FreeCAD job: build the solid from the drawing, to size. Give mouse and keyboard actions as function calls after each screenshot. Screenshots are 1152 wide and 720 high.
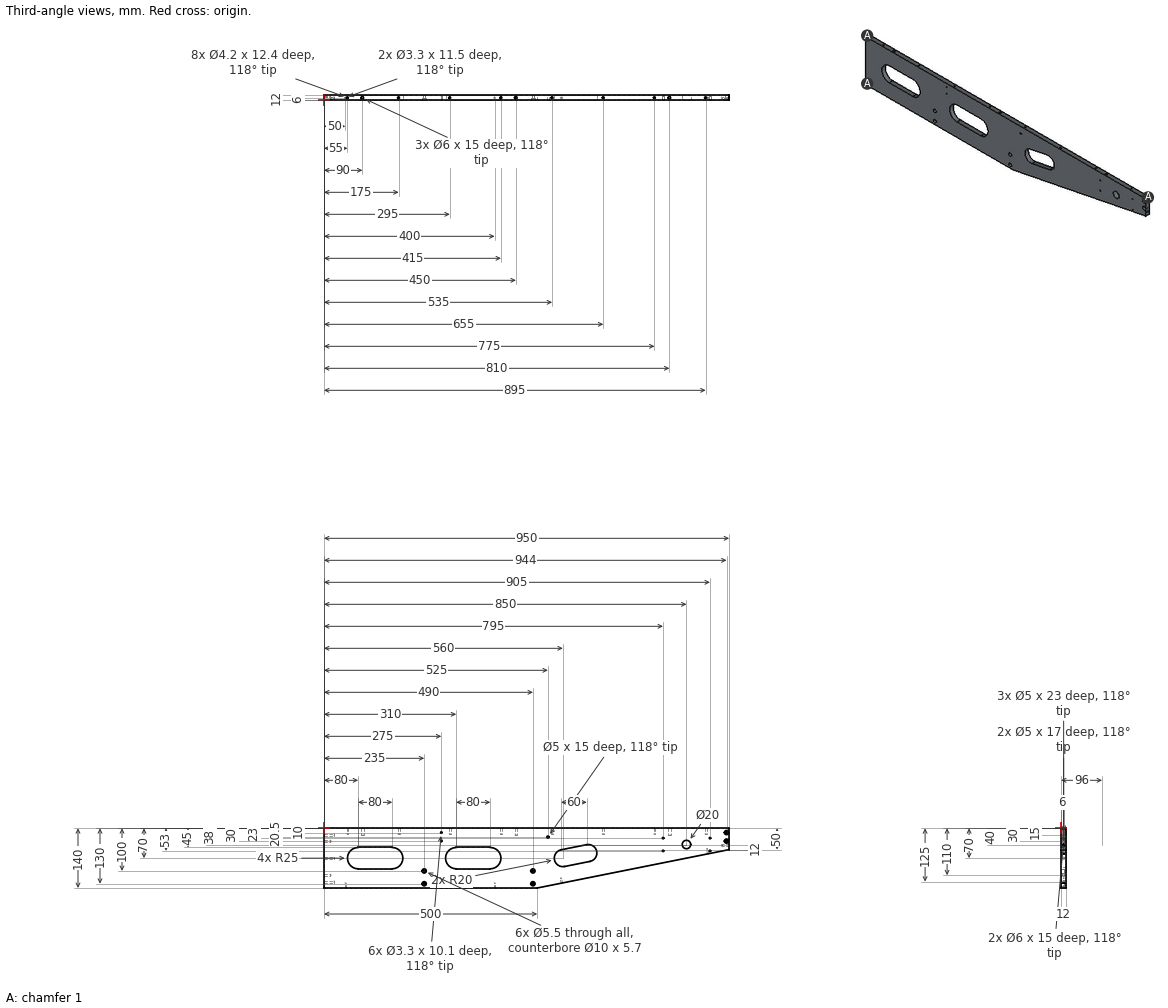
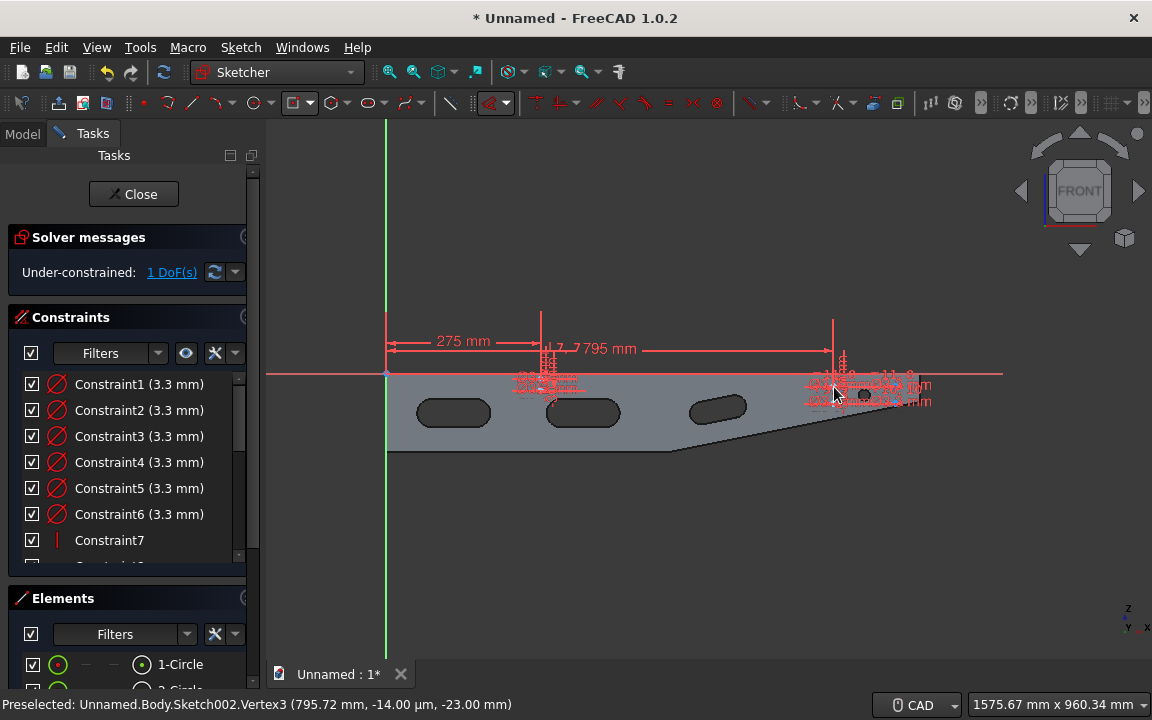
scroll(895, 387, up, 4)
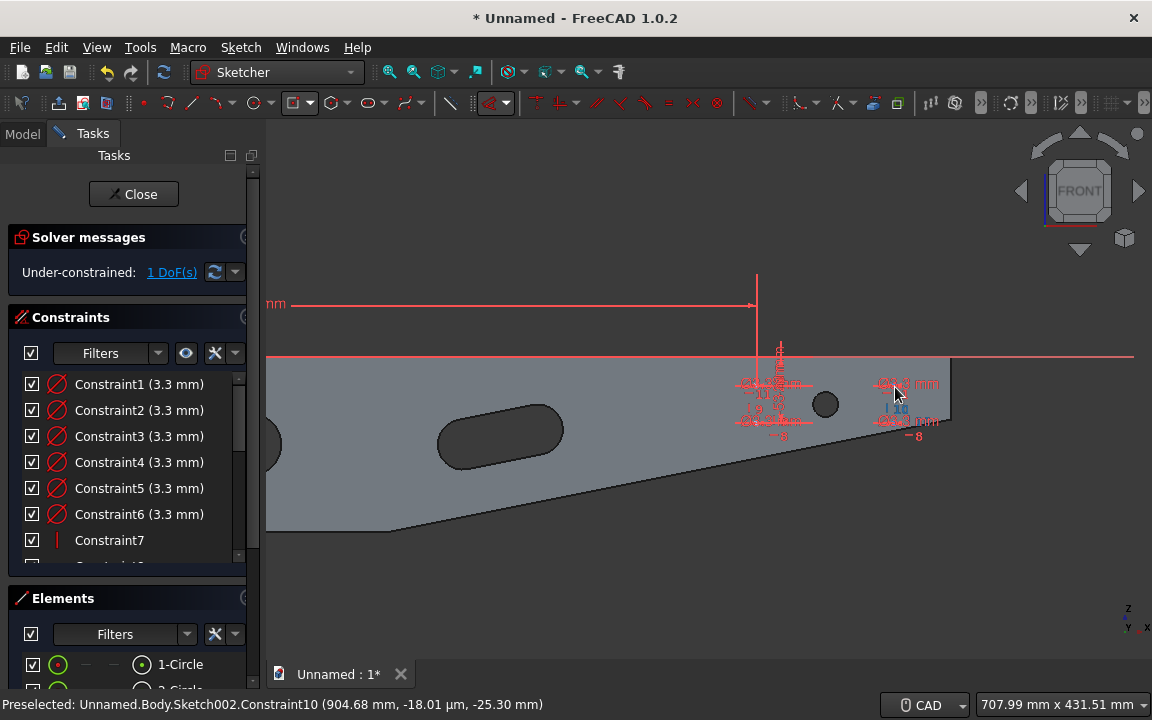
click(892, 384)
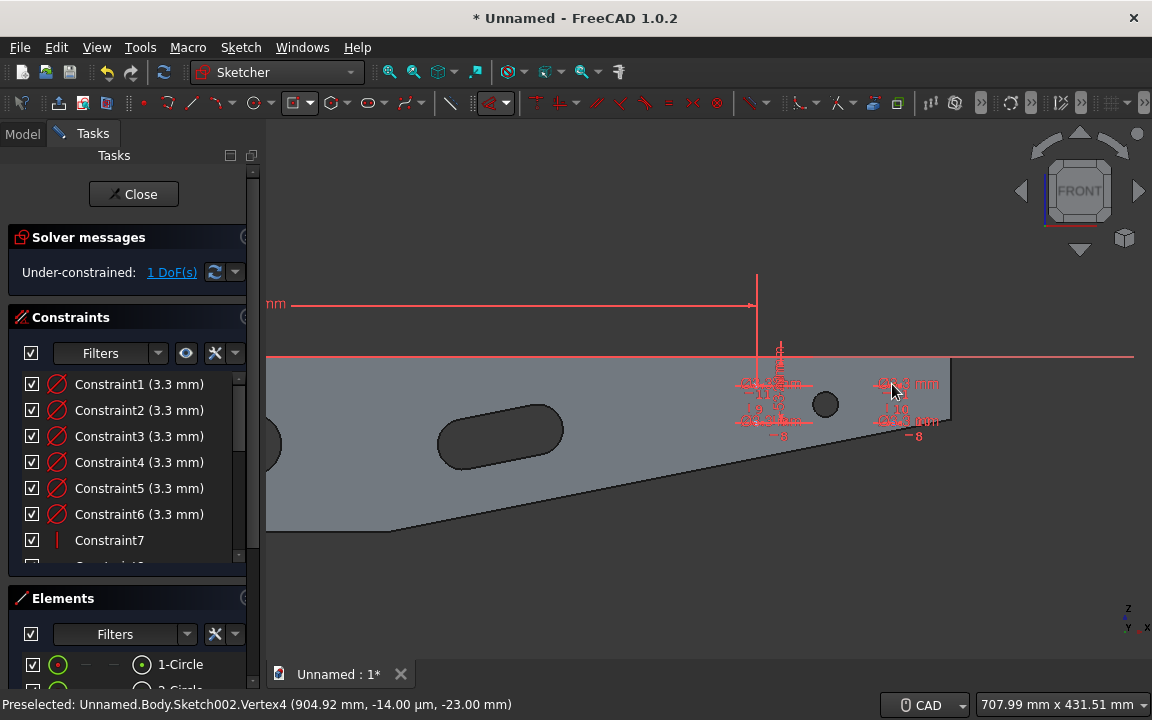
key(l)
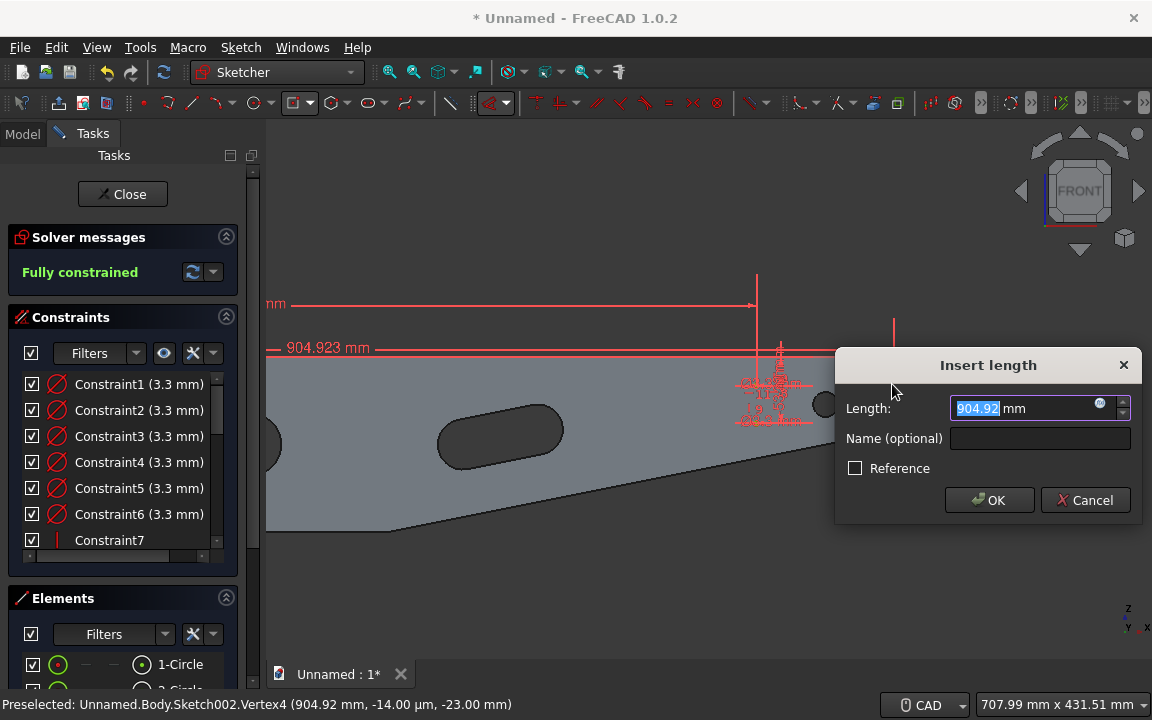
text(905)
key(Return)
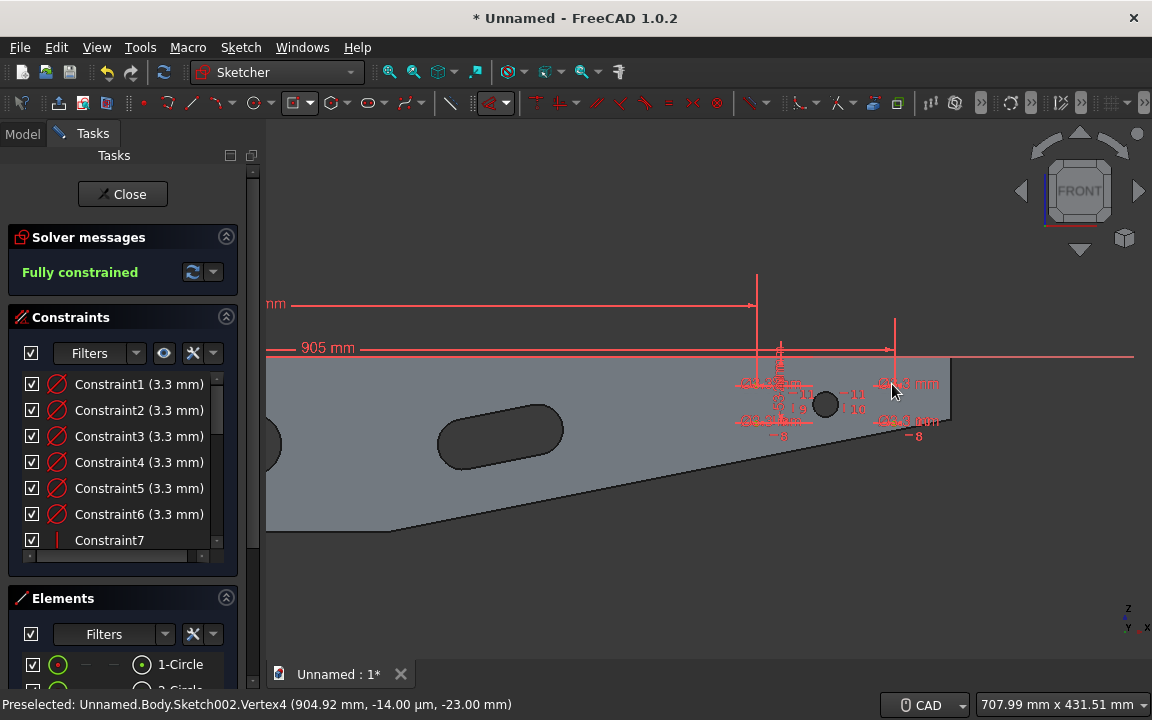
click(123, 194)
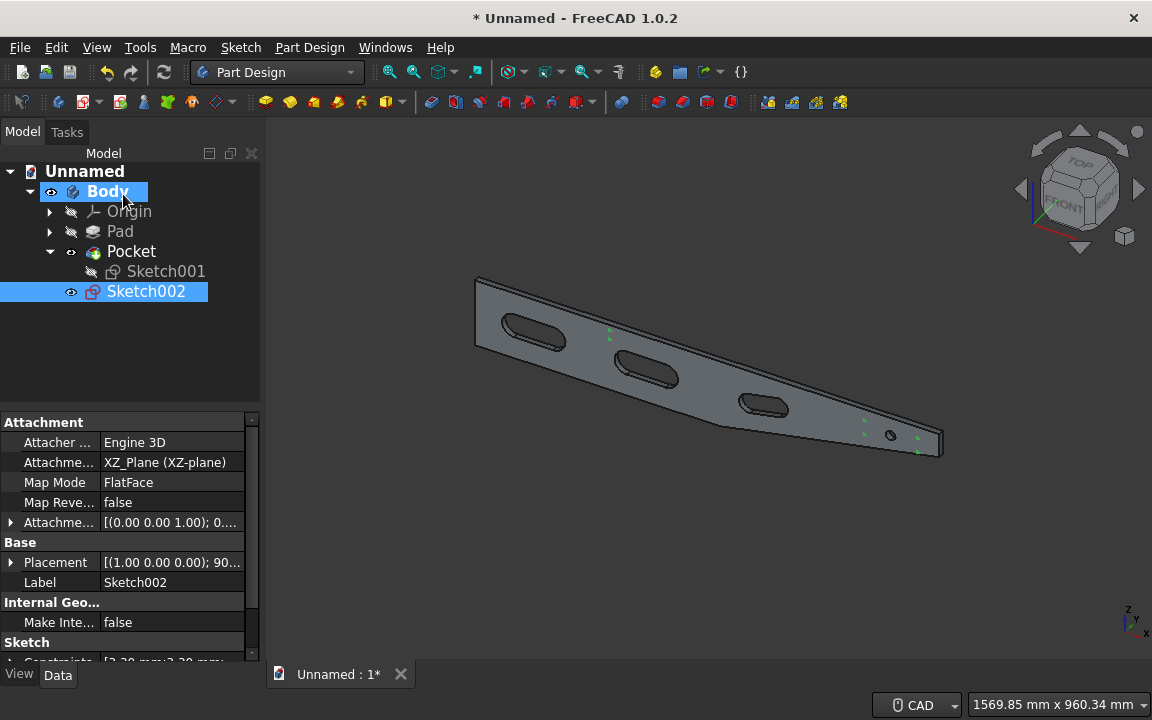
click(456, 102)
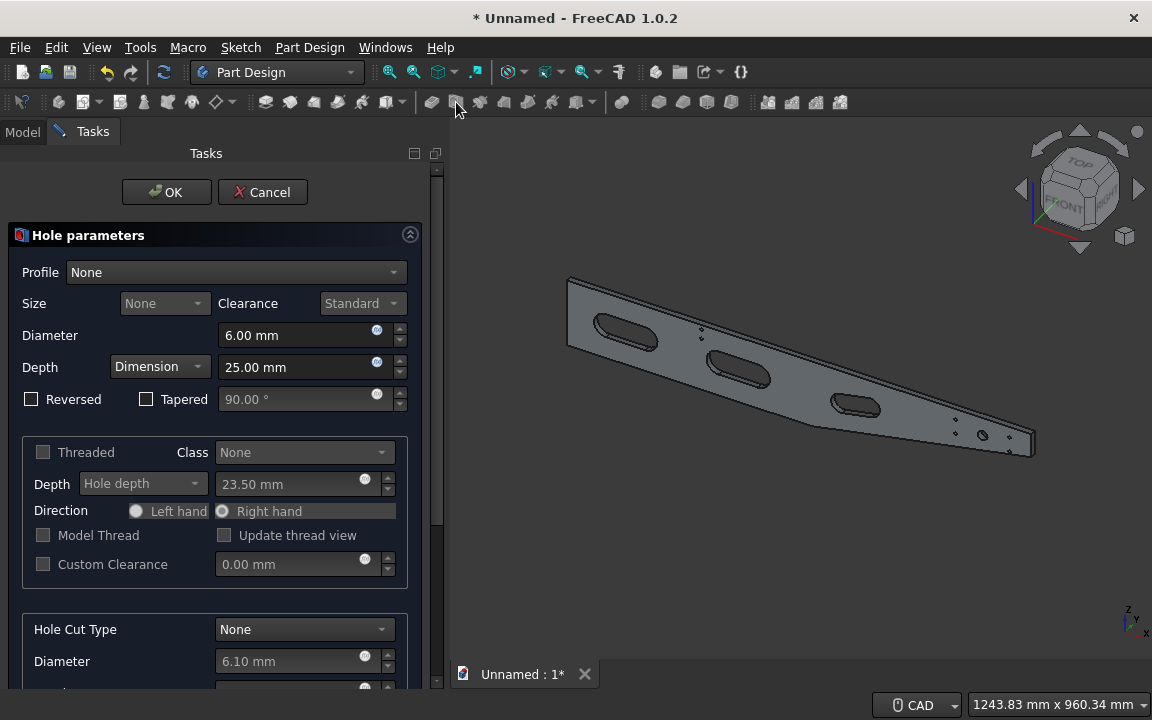
triple_click(305, 335)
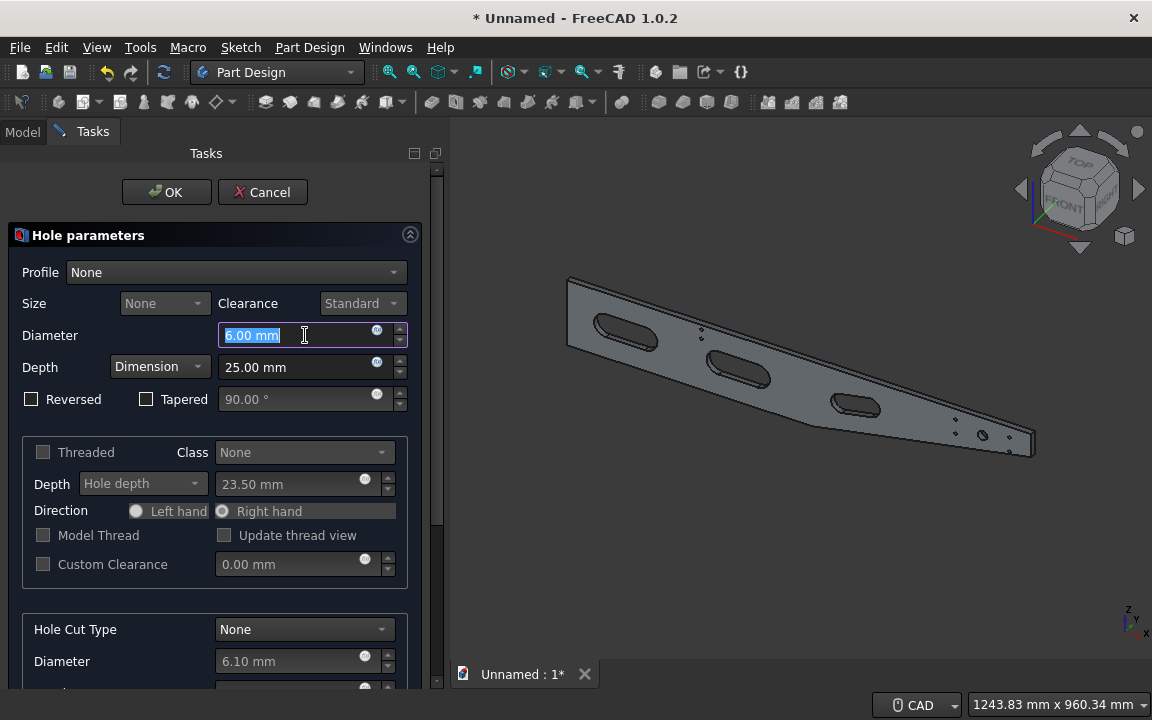
text(3.3)
key(Tab)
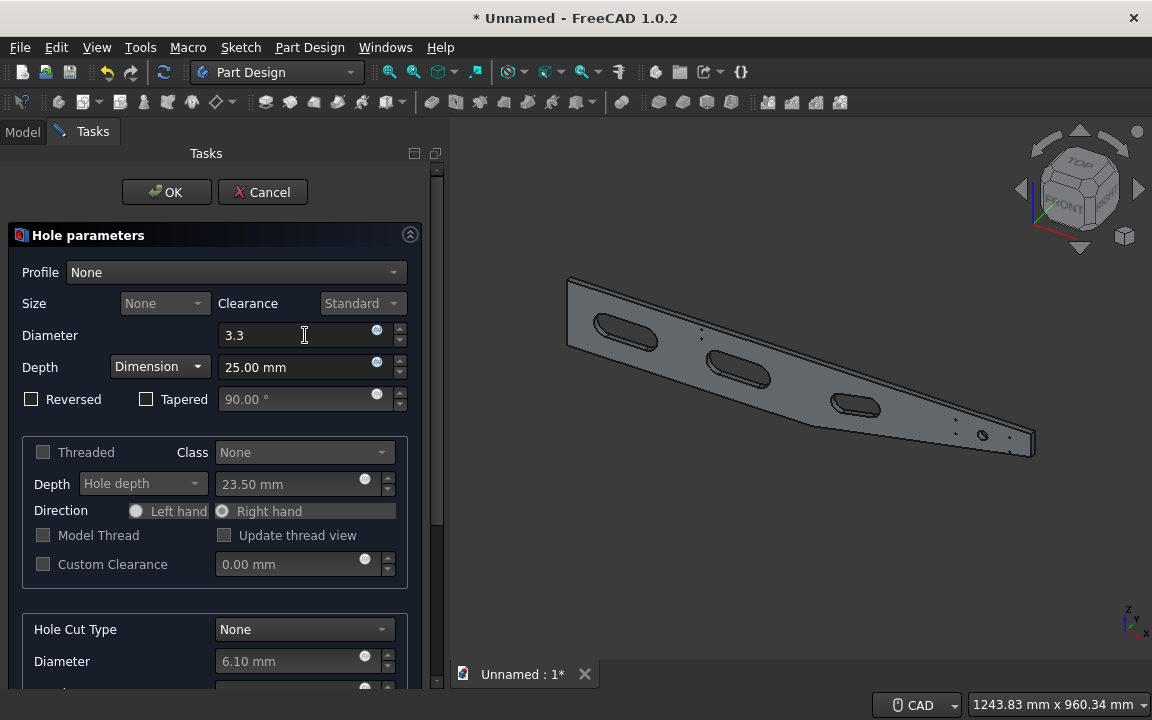
triple_click(305, 367)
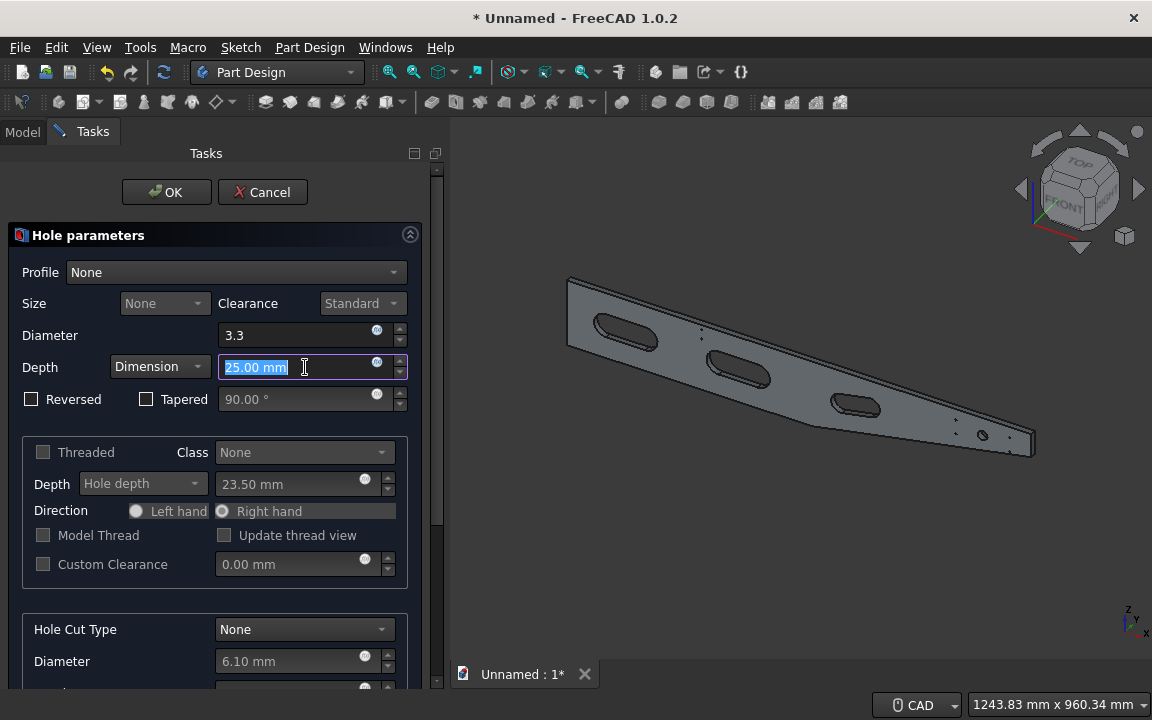
text(10.1)
key(Tab)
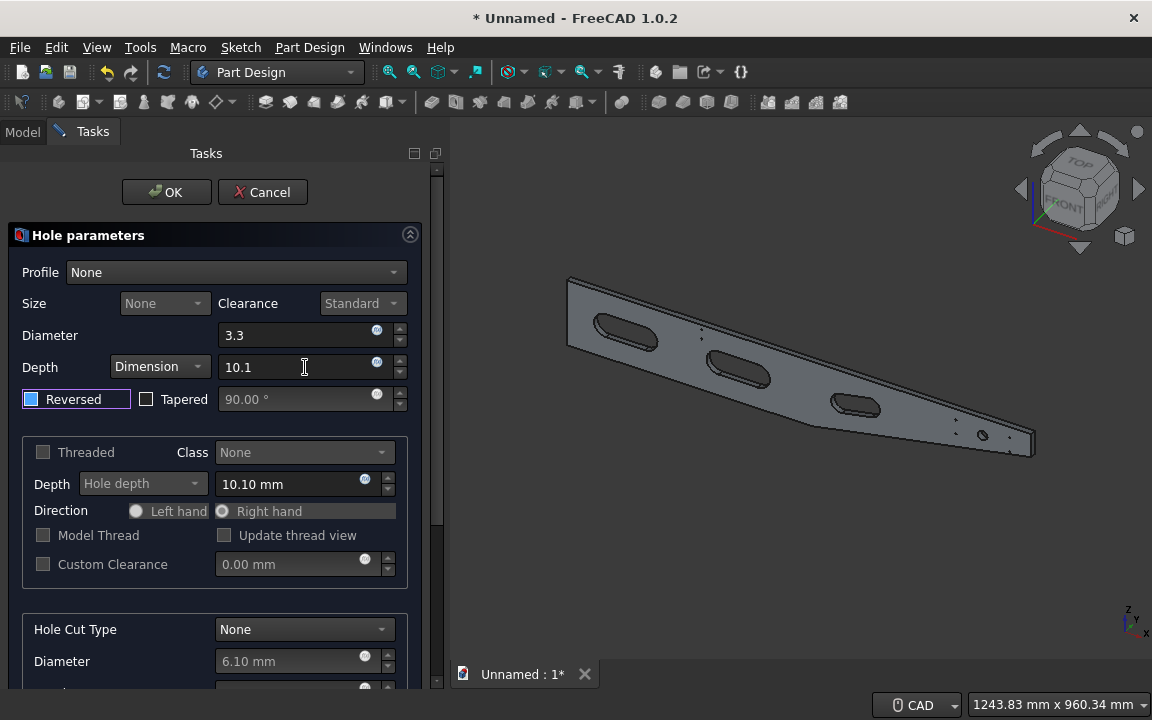
click(167, 192)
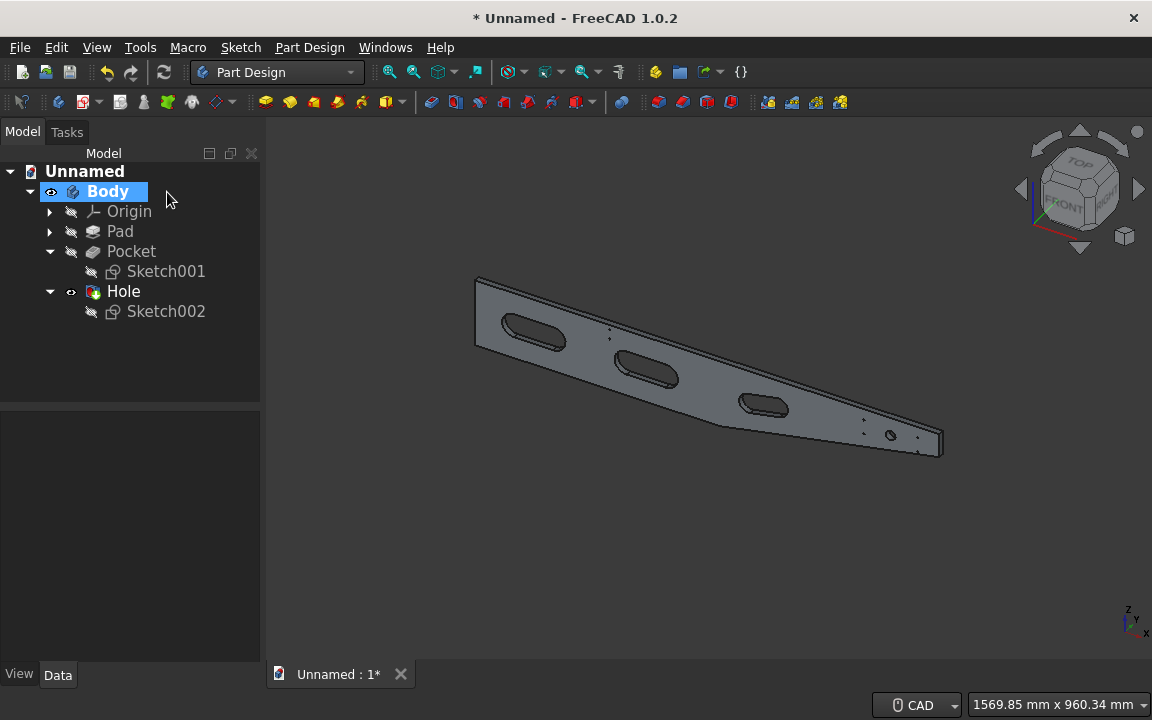
click(707, 389)